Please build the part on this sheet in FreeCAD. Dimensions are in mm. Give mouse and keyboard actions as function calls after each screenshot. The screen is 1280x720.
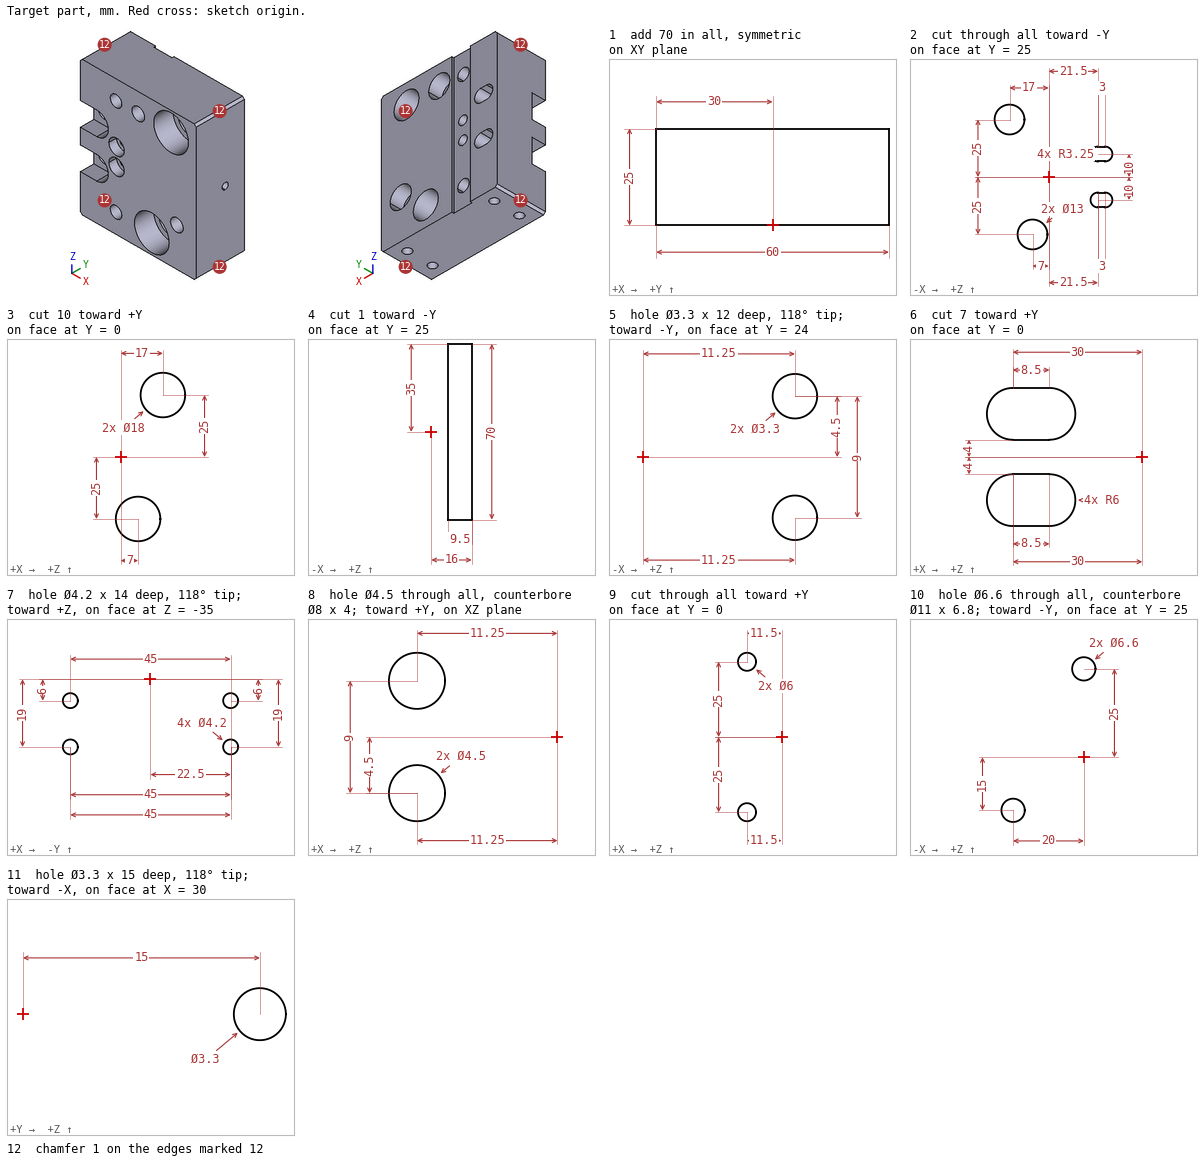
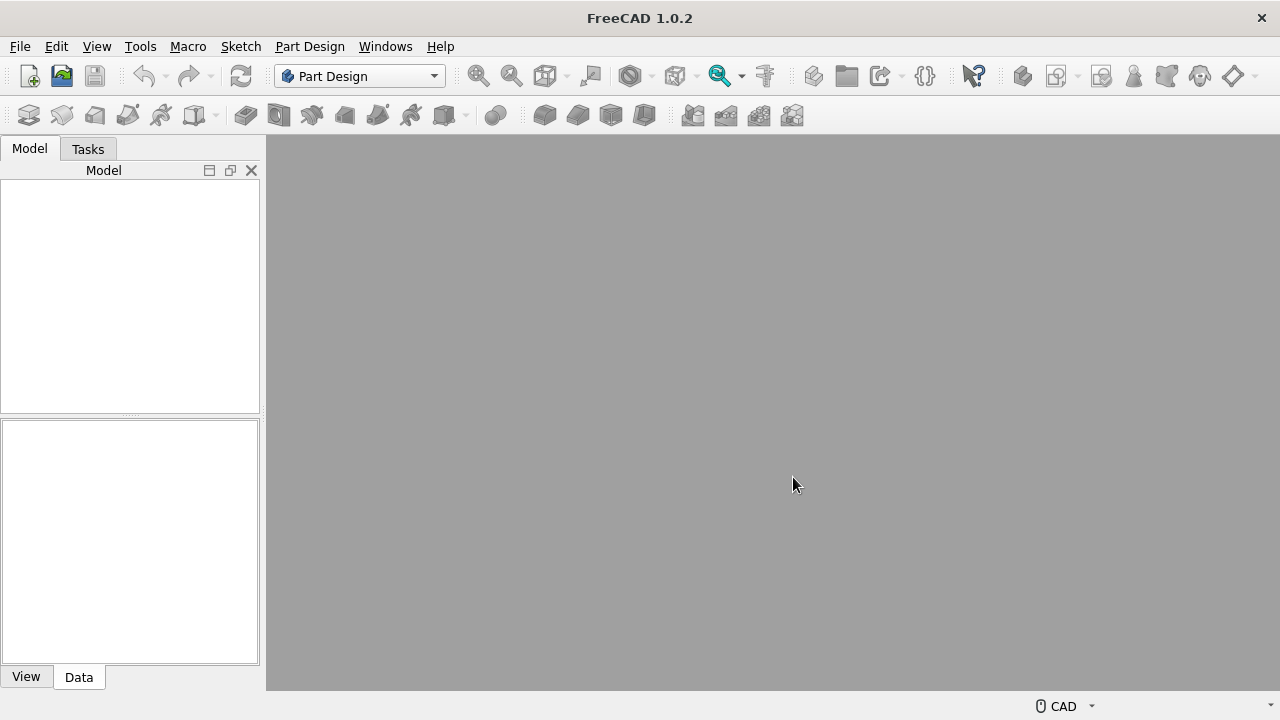
key(ctrl+n)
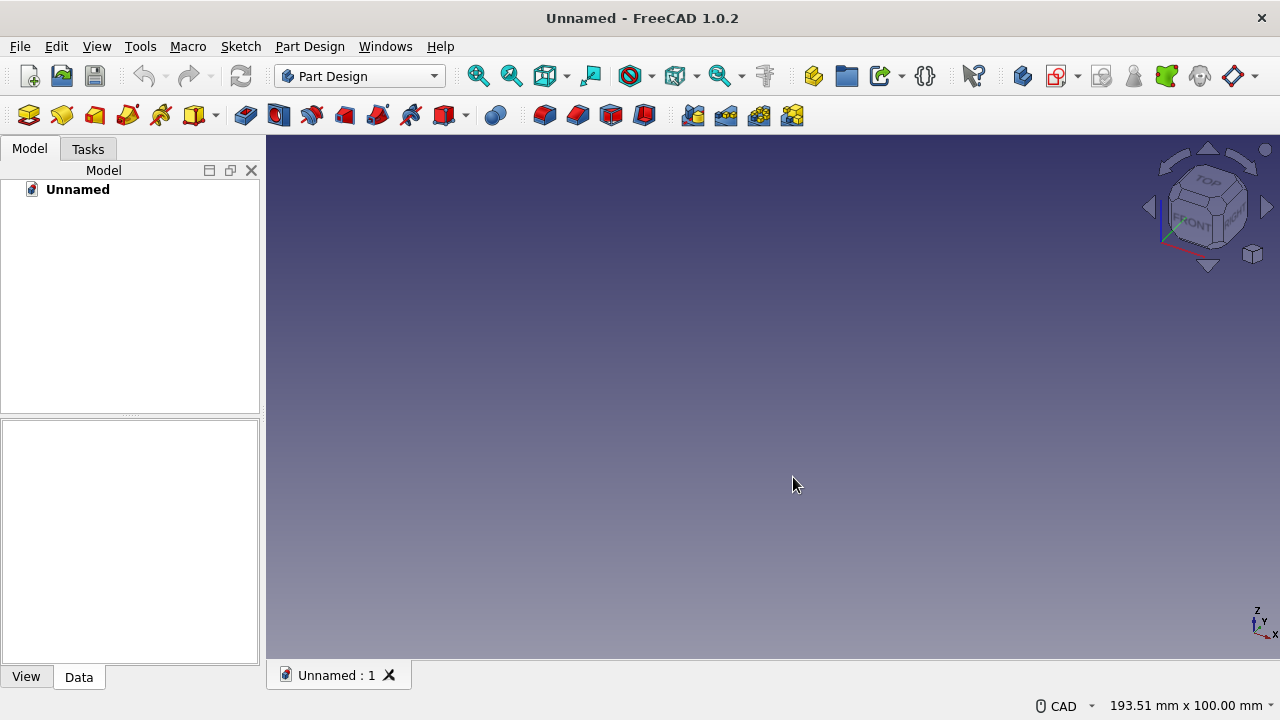
click(1056, 76)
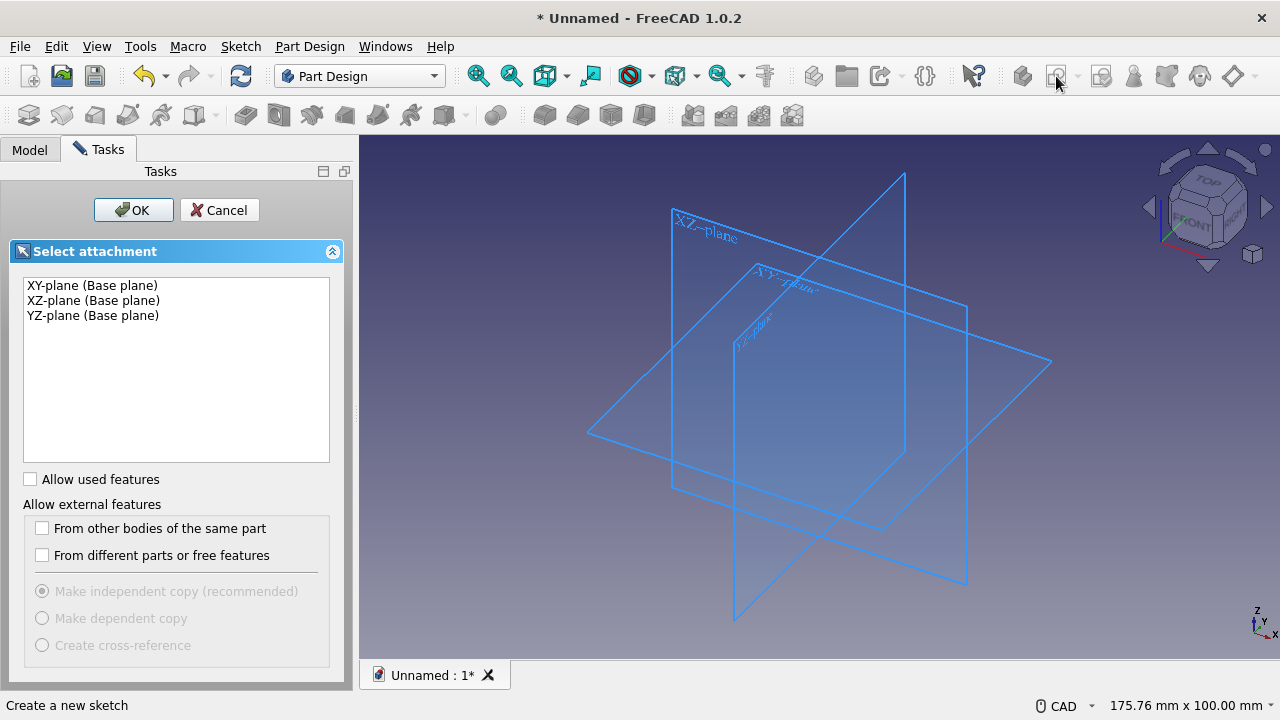
click(84, 286)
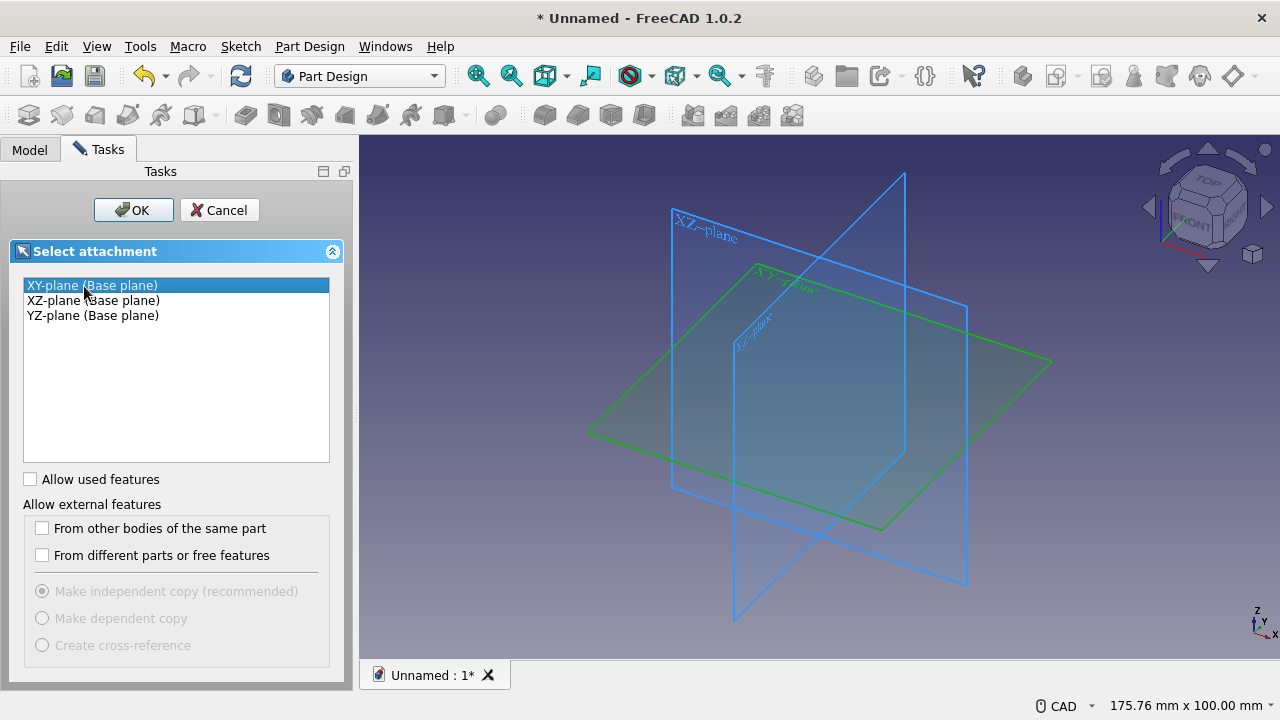
click(134, 210)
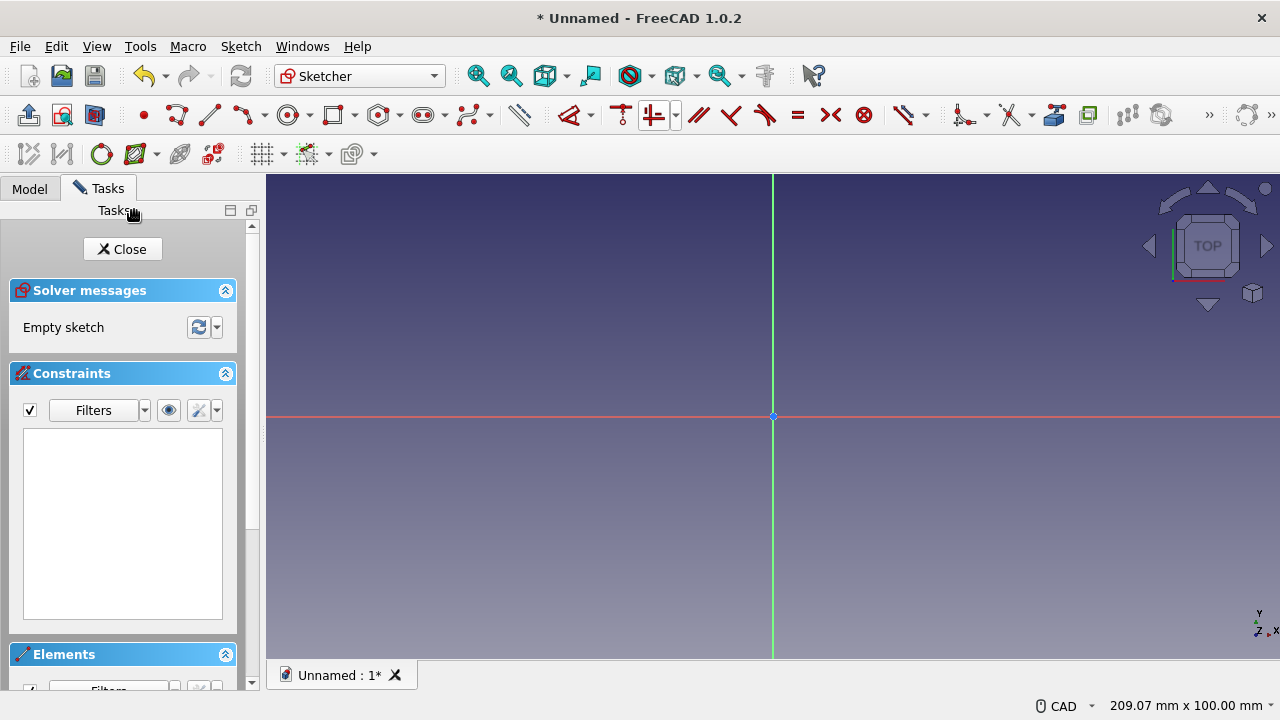
scroll(856, 282, up, 3)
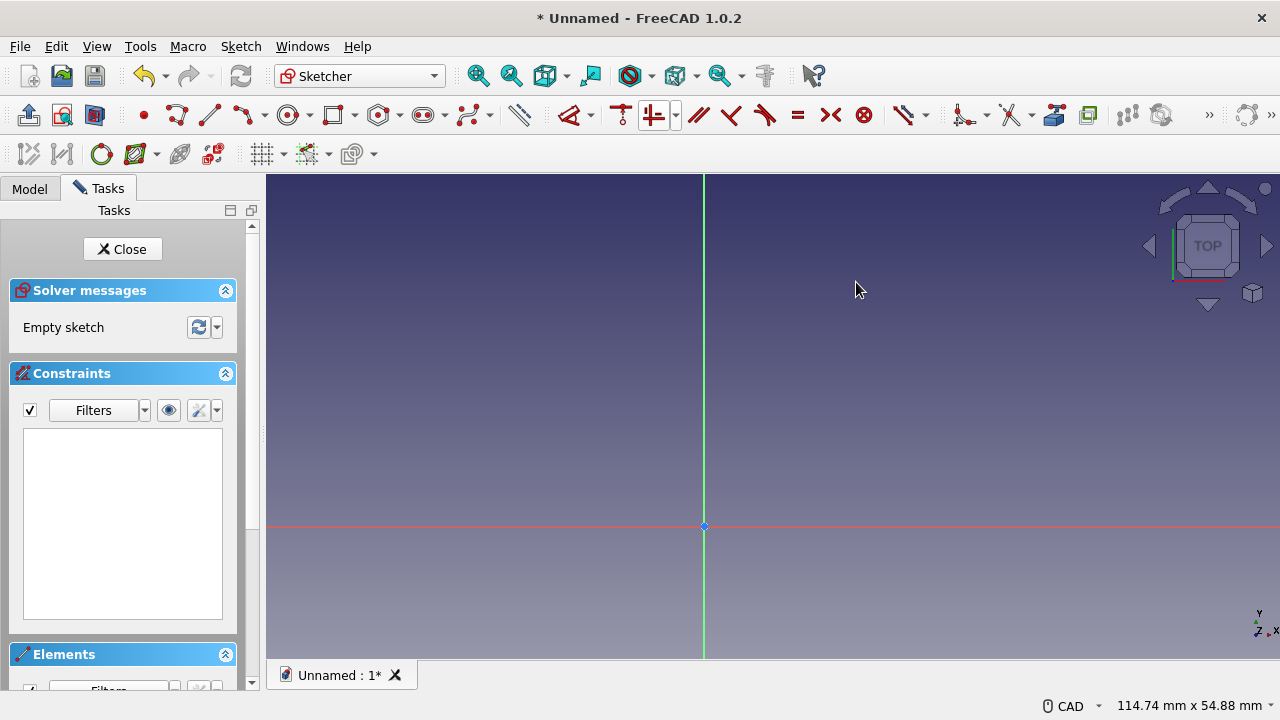
key(g)
key(r)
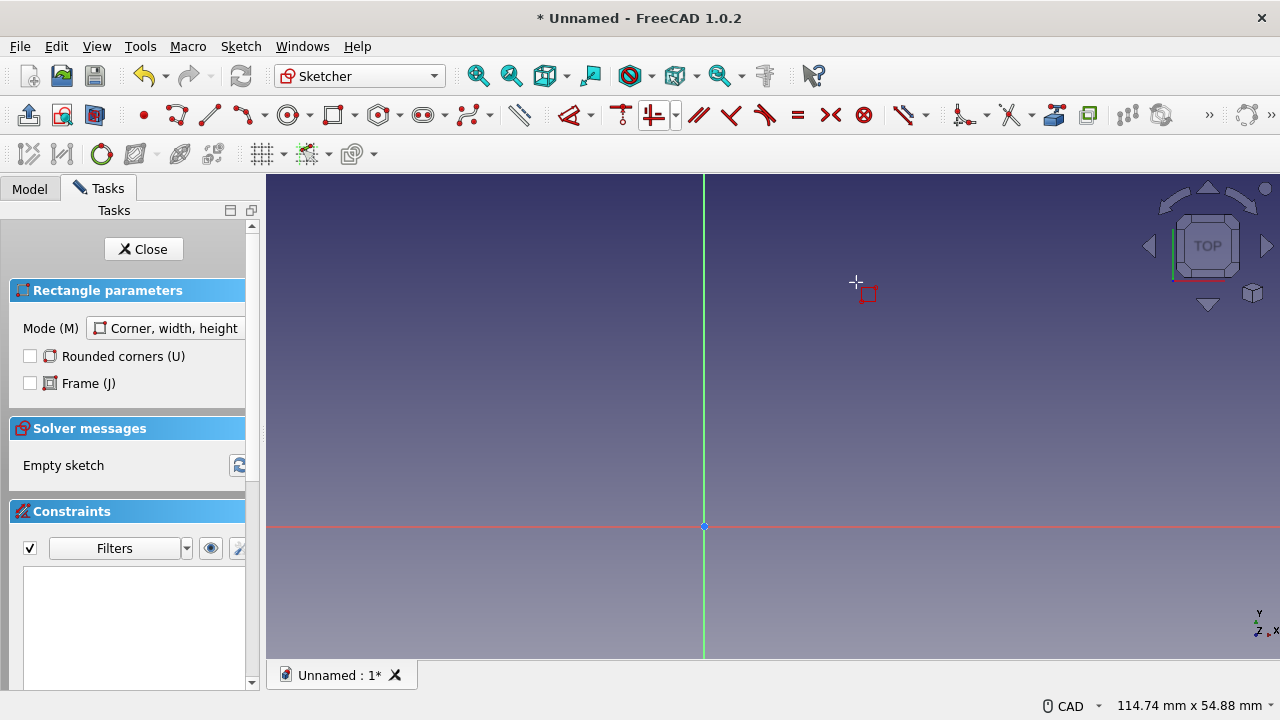
click(439, 306)
click(969, 527)
key(Escape)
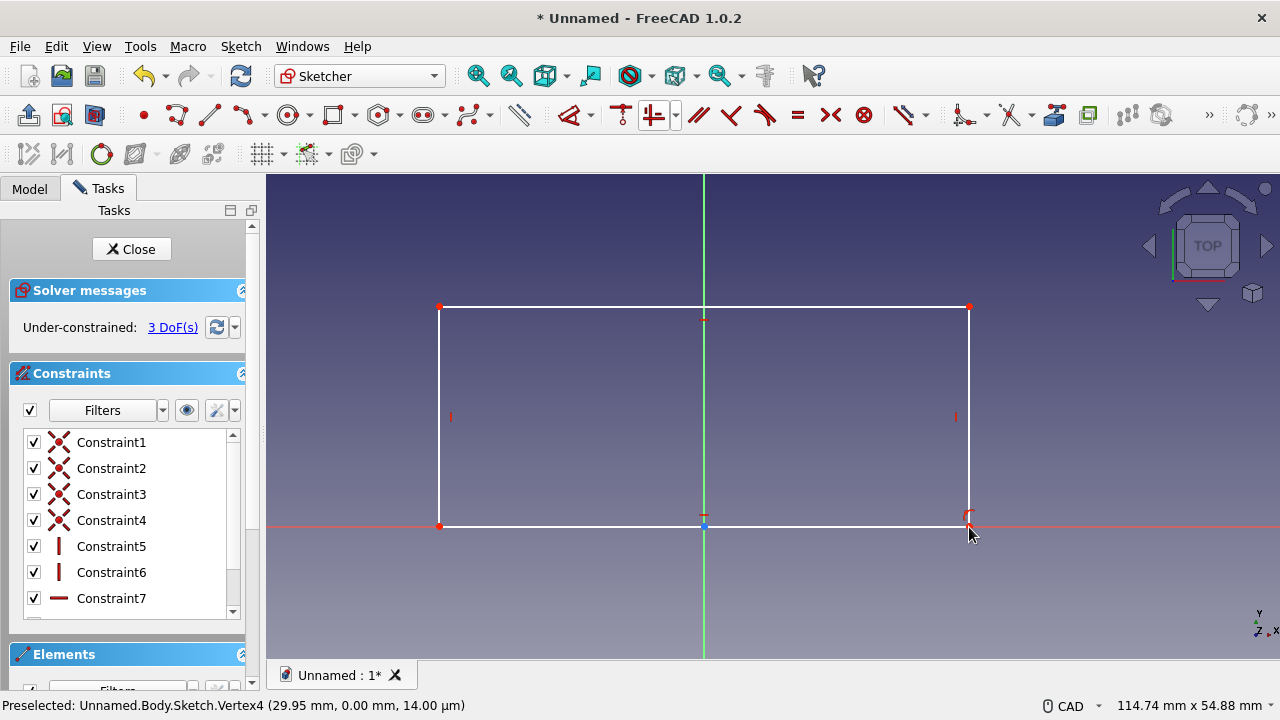
key(d)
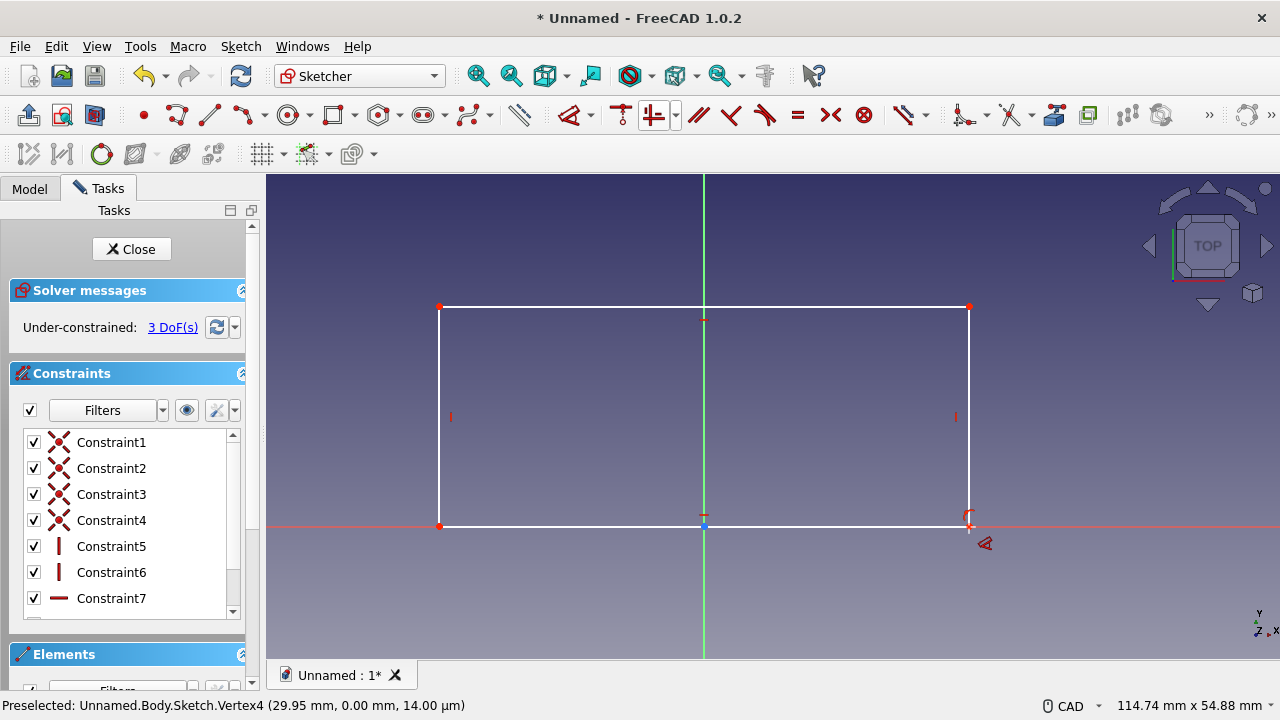
click(439, 373)
click(405, 417)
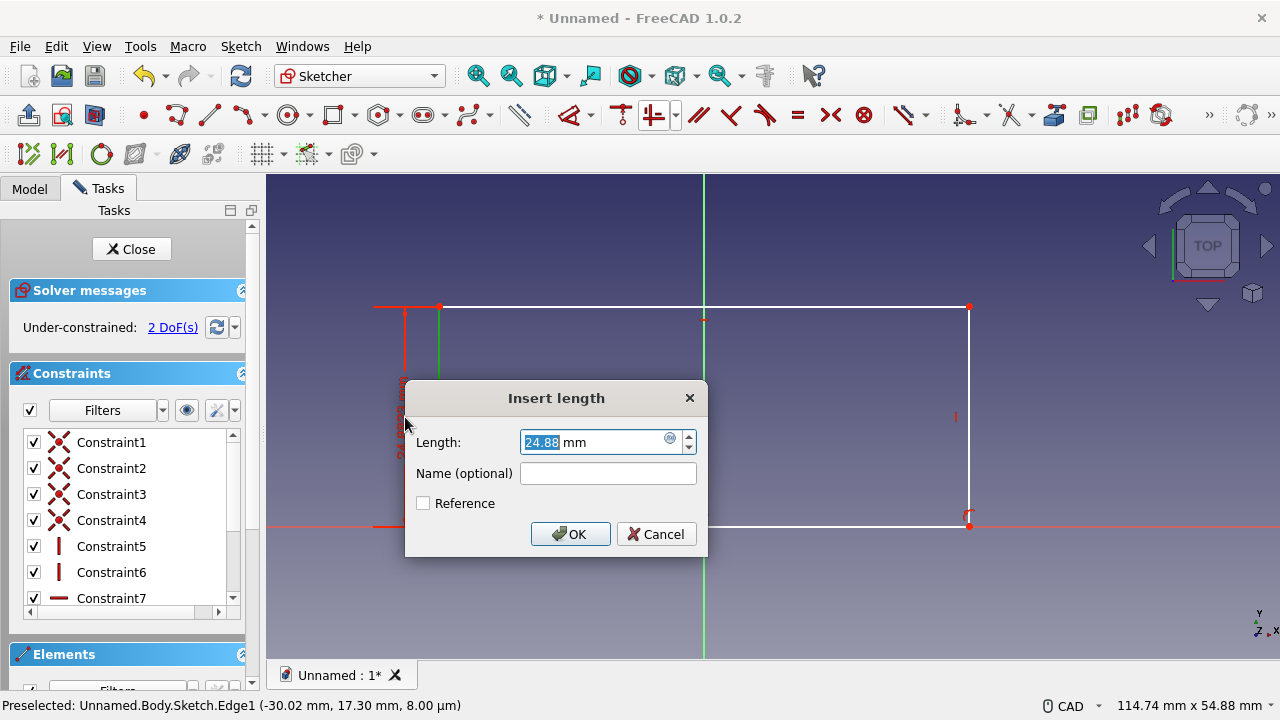
text(25)
key(Return)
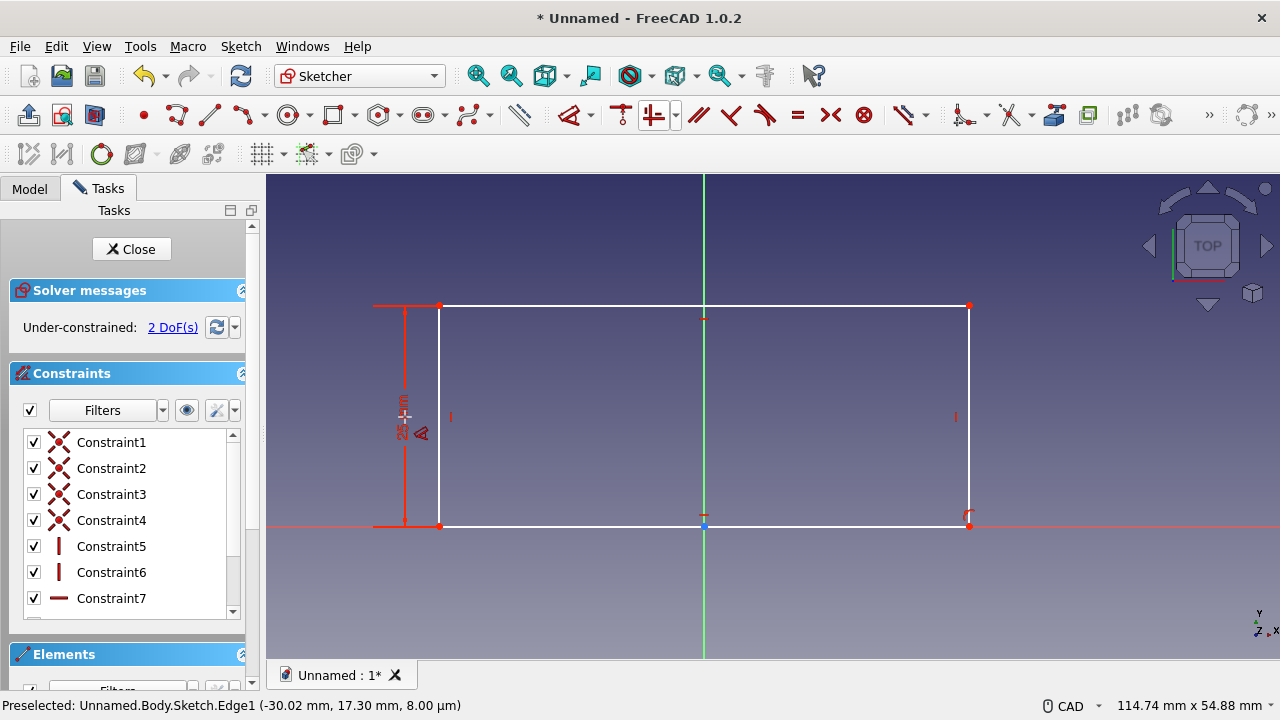
click(598, 527)
click(582, 561)